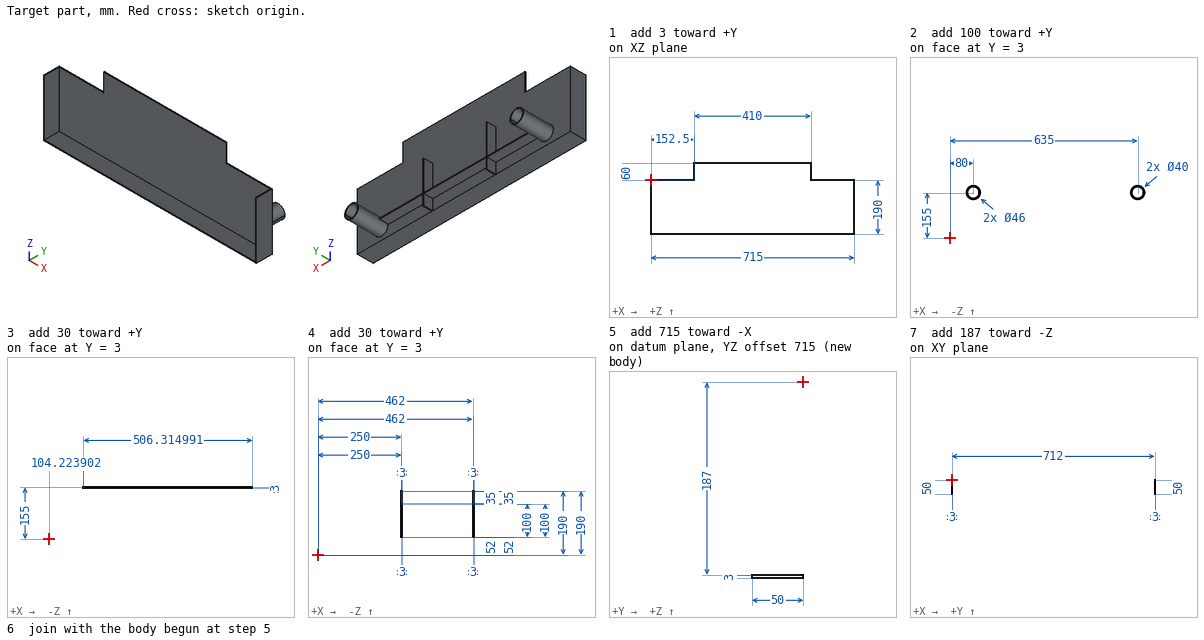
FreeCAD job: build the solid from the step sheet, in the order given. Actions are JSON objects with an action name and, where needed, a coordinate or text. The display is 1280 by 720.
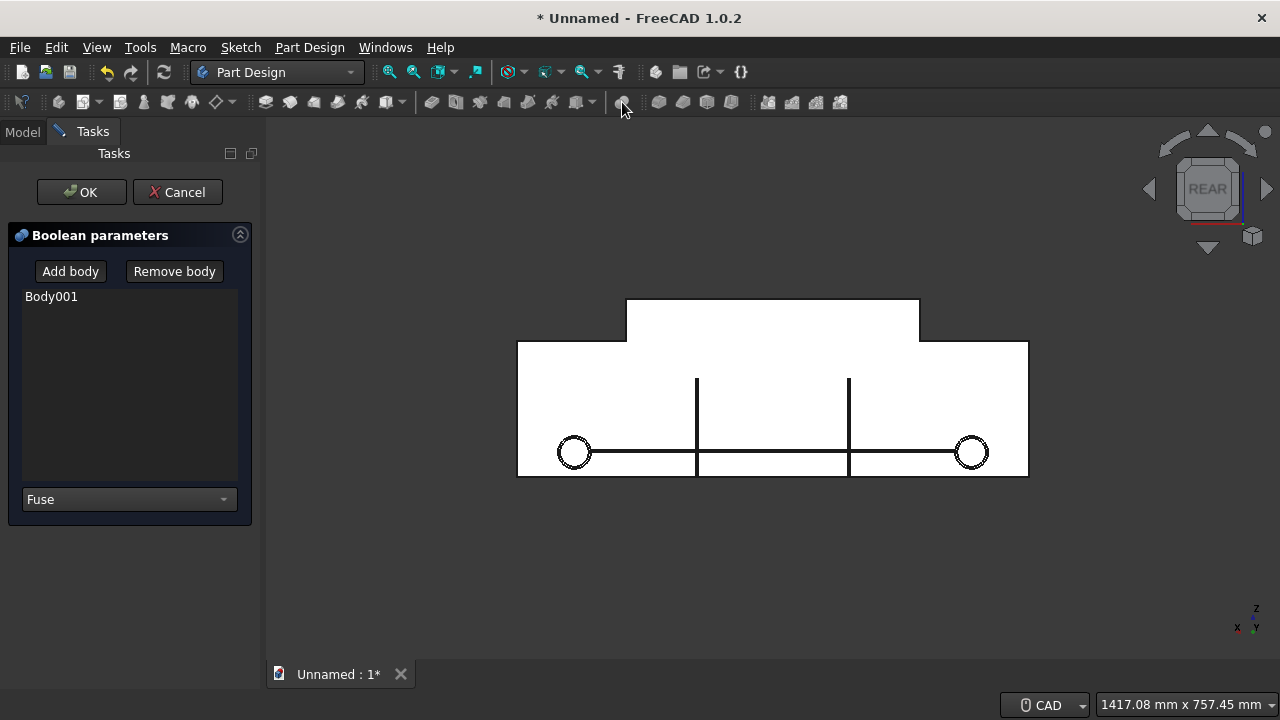
{"action": "left_click", "coordinate": [82, 192]}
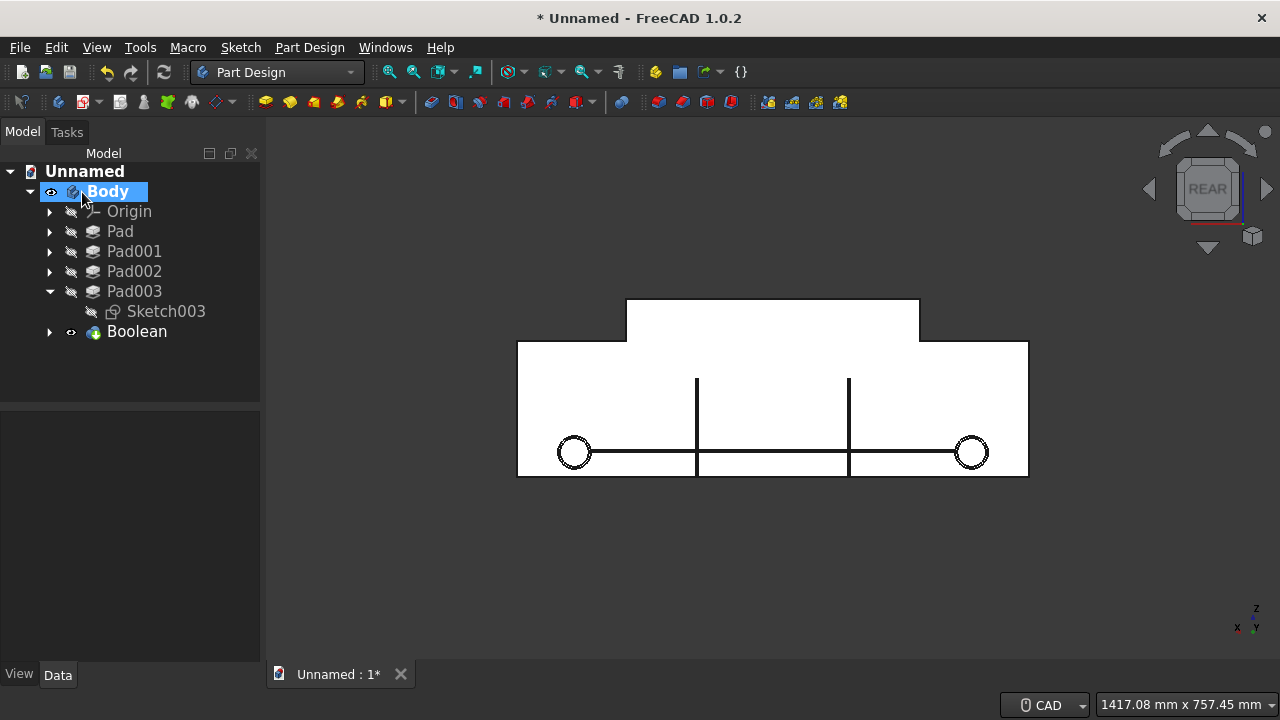
{"action": "left_click", "coordinate": [84, 102]}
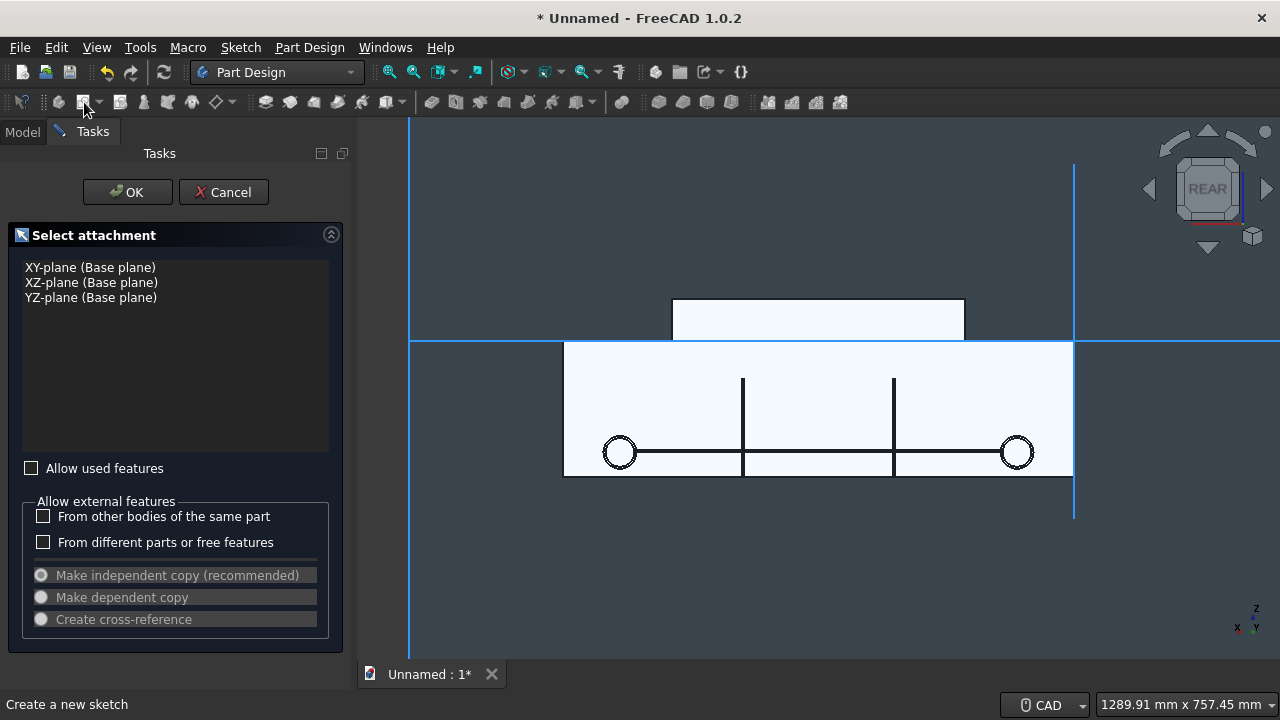
{"action": "left_click", "coordinate": [82, 268]}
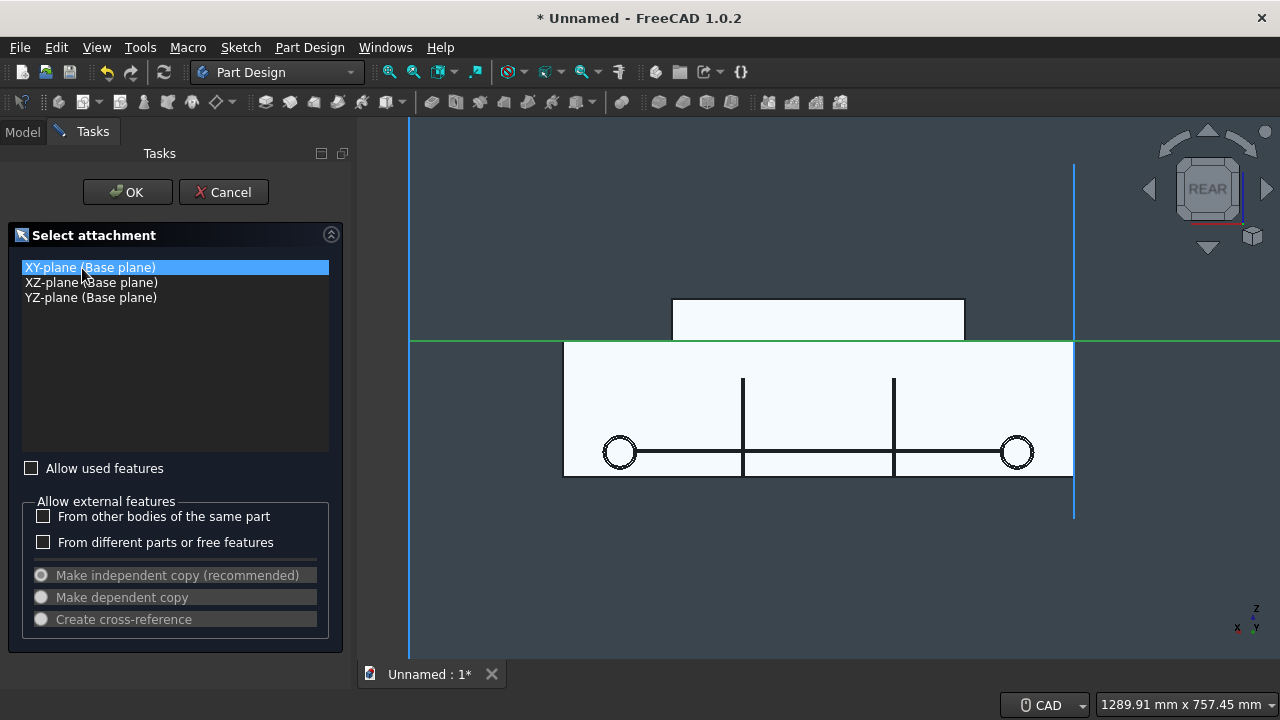
{"action": "left_click", "coordinate": [128, 192]}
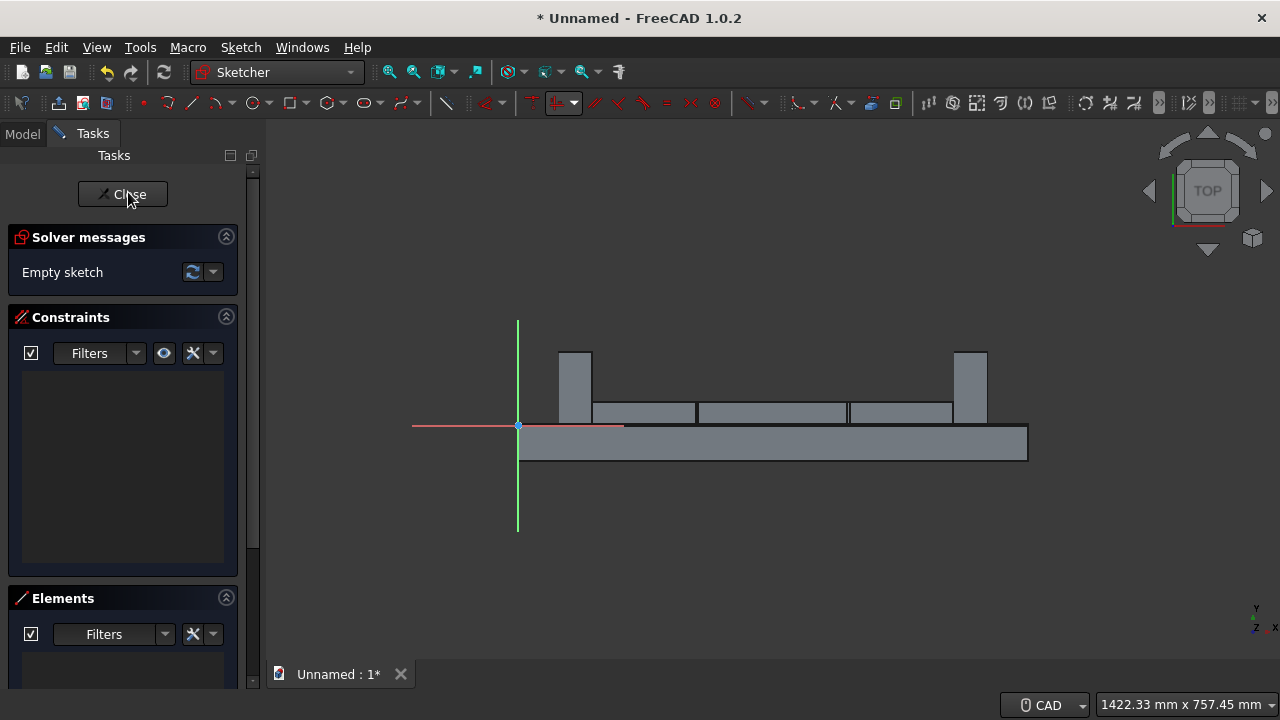
{"action": "left_click", "coordinate": [108, 104]}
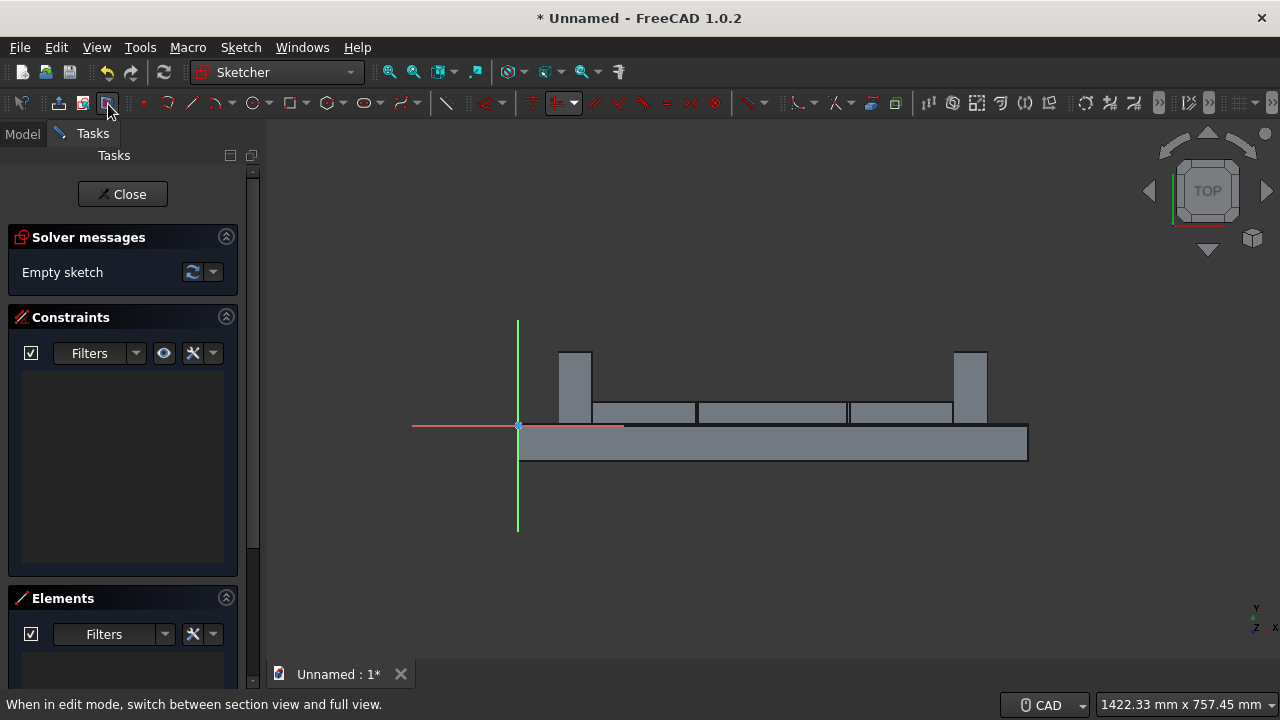
{"action": "left_click", "coordinate": [290, 104]}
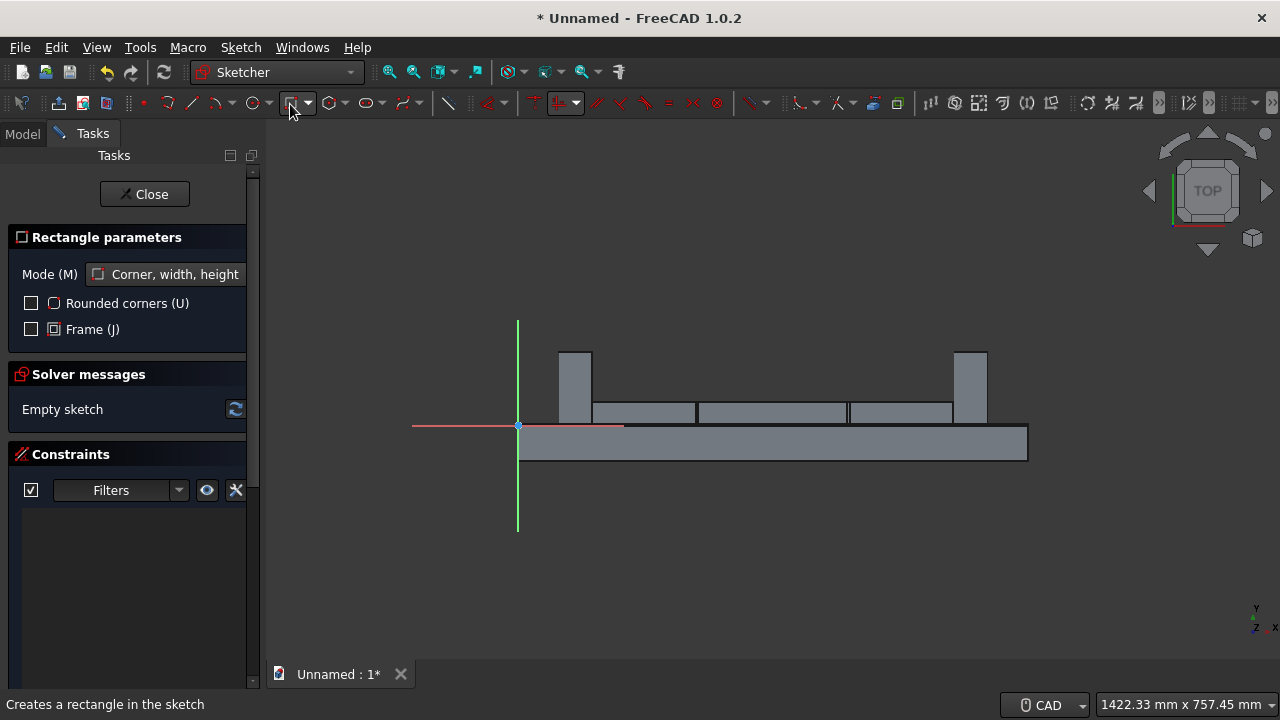
{"action": "scroll", "coordinate": [1026, 426], "scroll_direction": "up", "scroll_amount": 11}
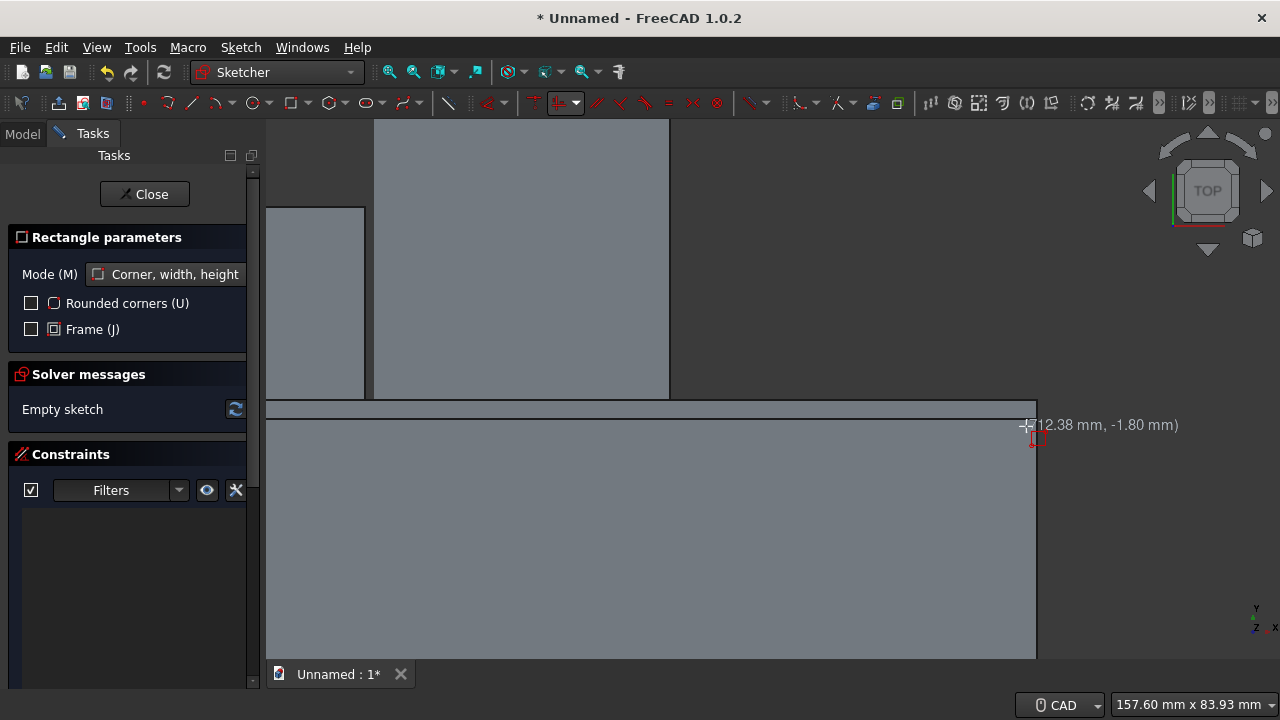
{"action": "scroll", "coordinate": [1013, 359], "scroll_direction": "down", "scroll_amount": 10}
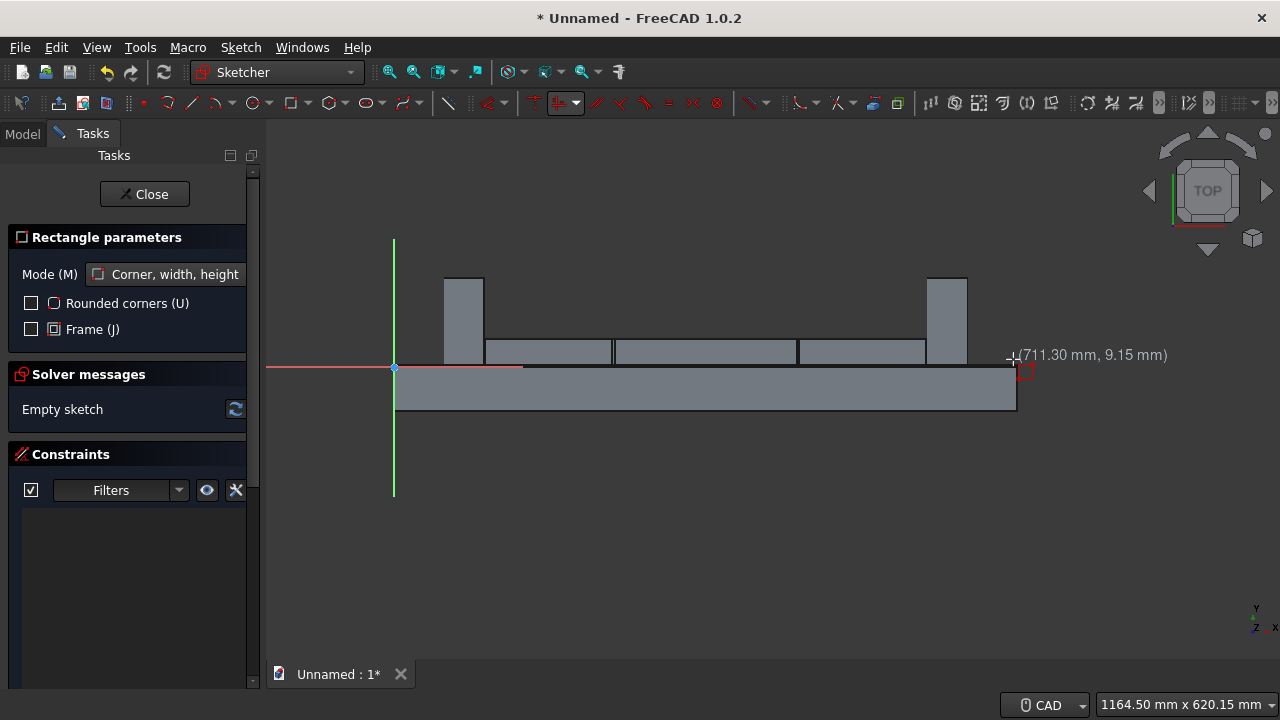
{"action": "left_click", "coordinate": [1014, 367]}
{"action": "mouse_move", "coordinate": [1017, 411]}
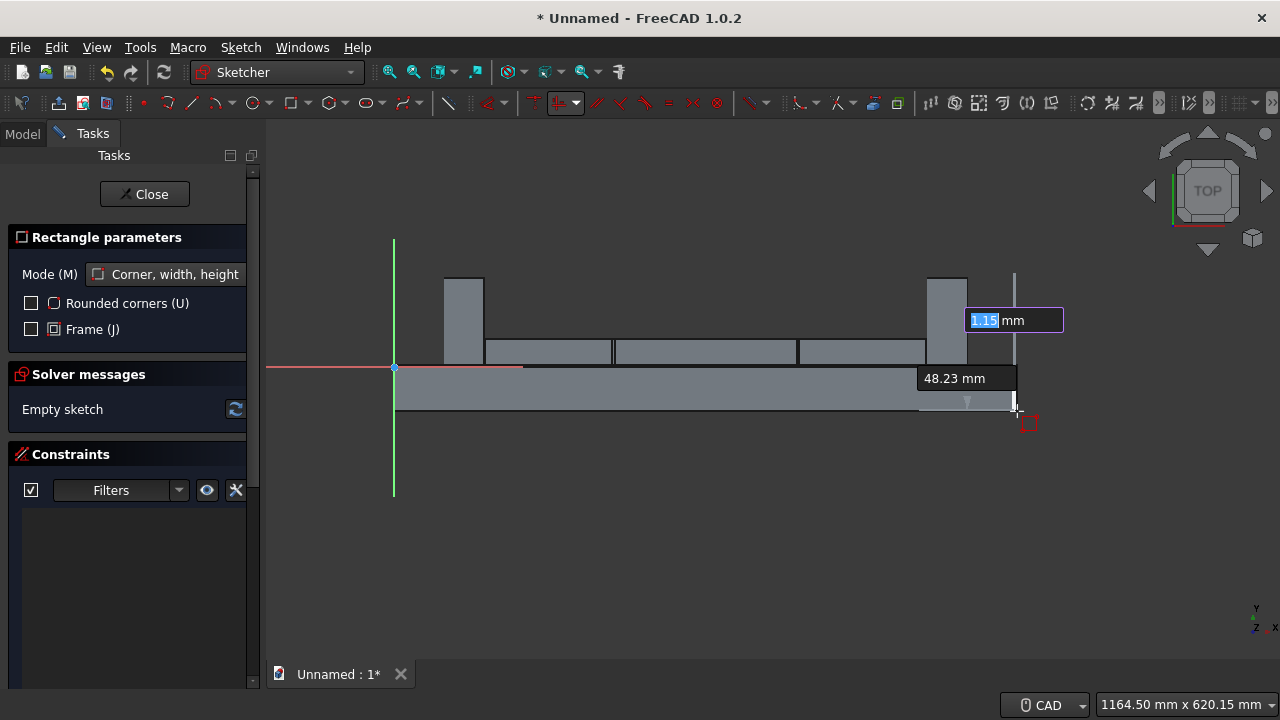
{"action": "type", "text": "3"}
{"action": "key", "text": "Tab"}
{"action": "type", "text": "50"}
{"action": "key", "text": "Return"}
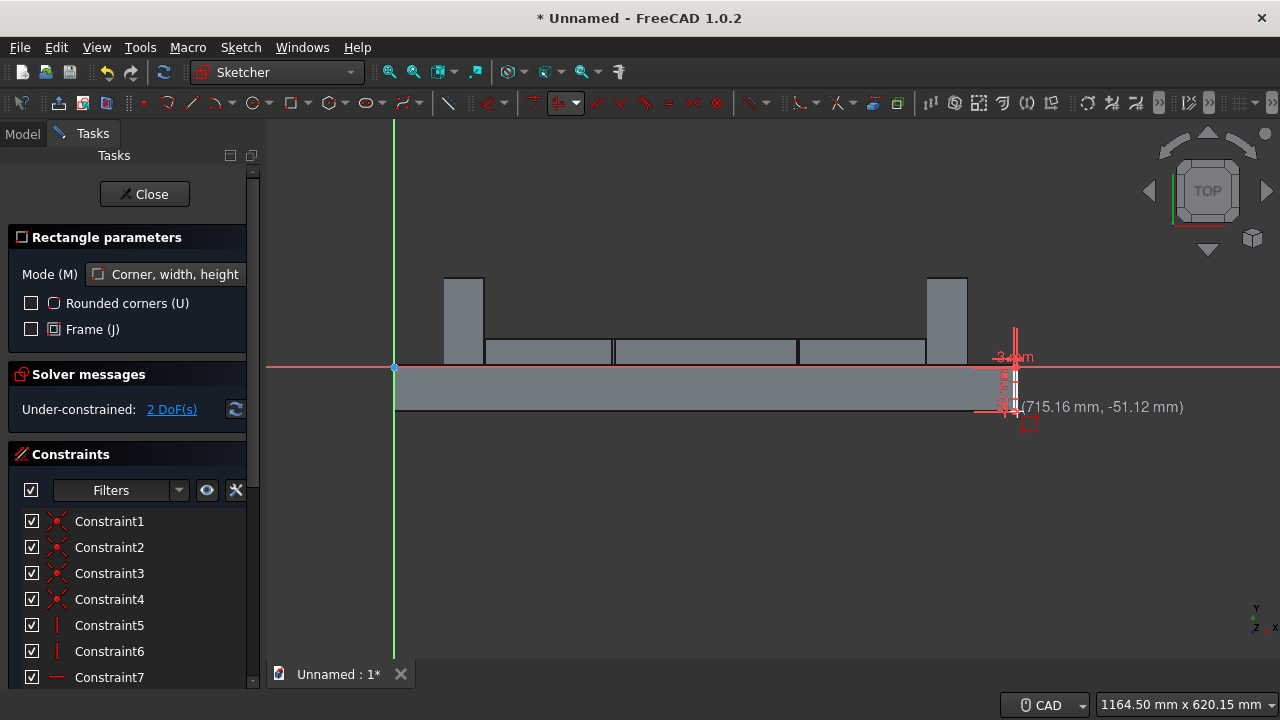
{"action": "scroll", "coordinate": [394, 367], "scroll_direction": "up", "scroll_amount": 10}